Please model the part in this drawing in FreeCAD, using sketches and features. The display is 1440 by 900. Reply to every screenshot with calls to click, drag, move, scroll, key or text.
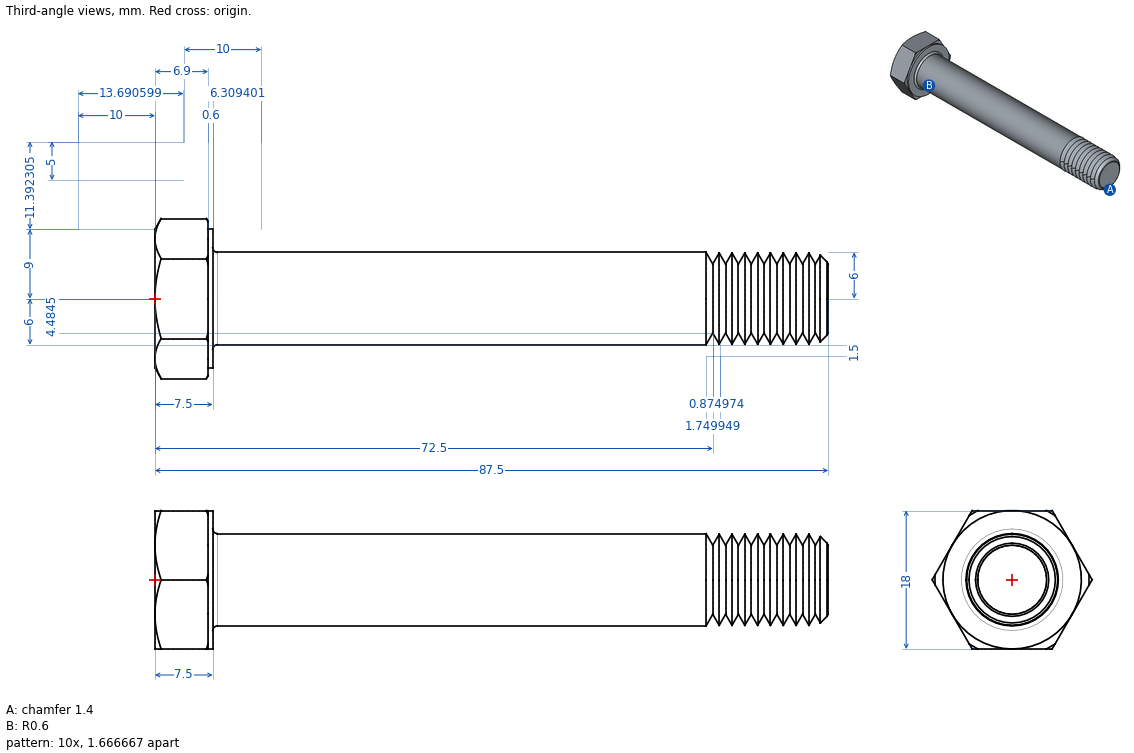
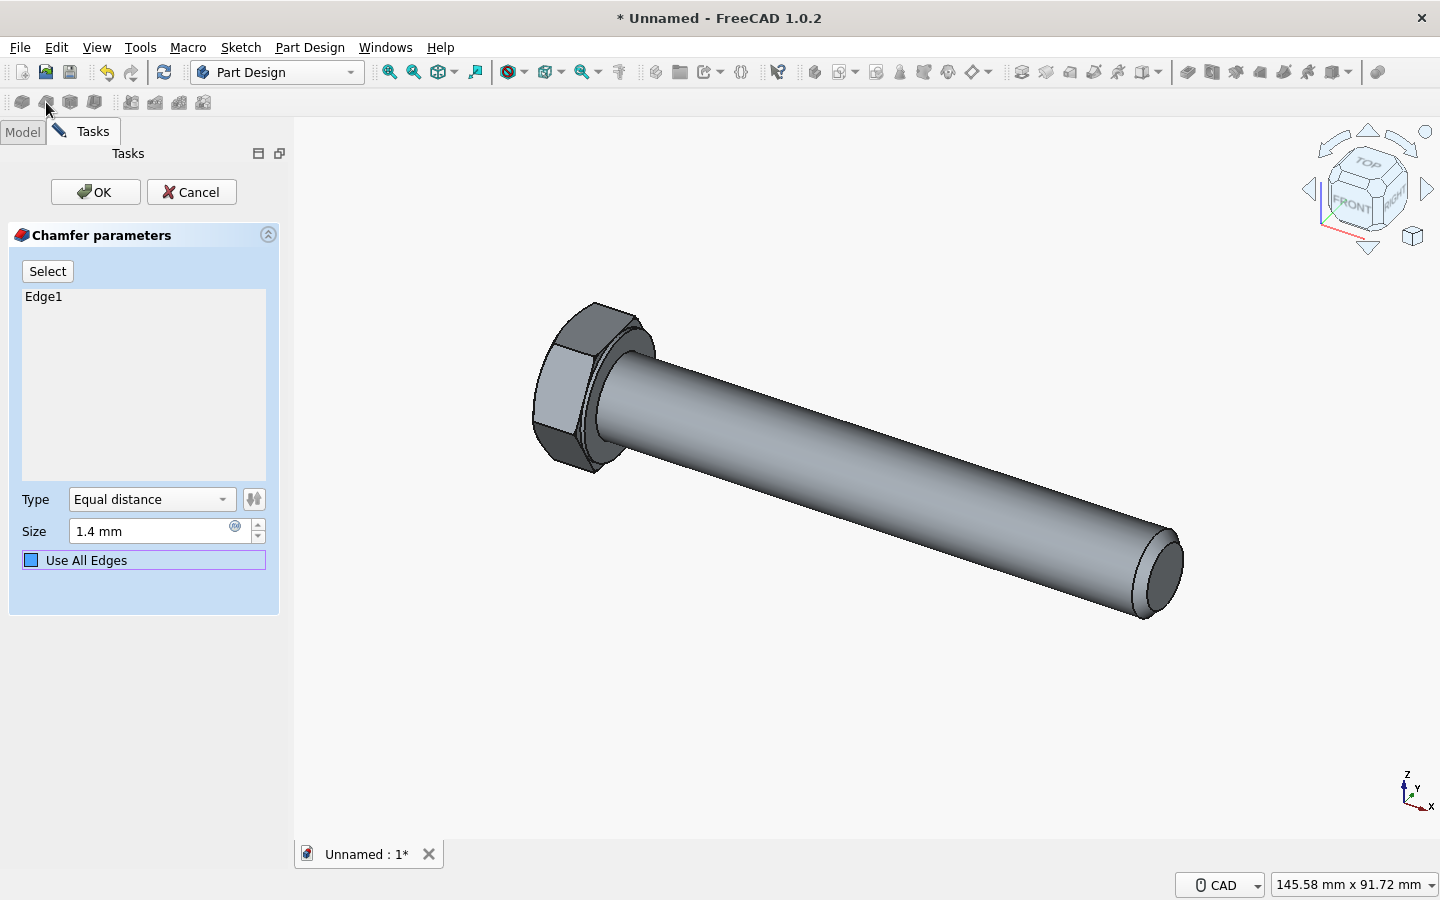
click(96, 192)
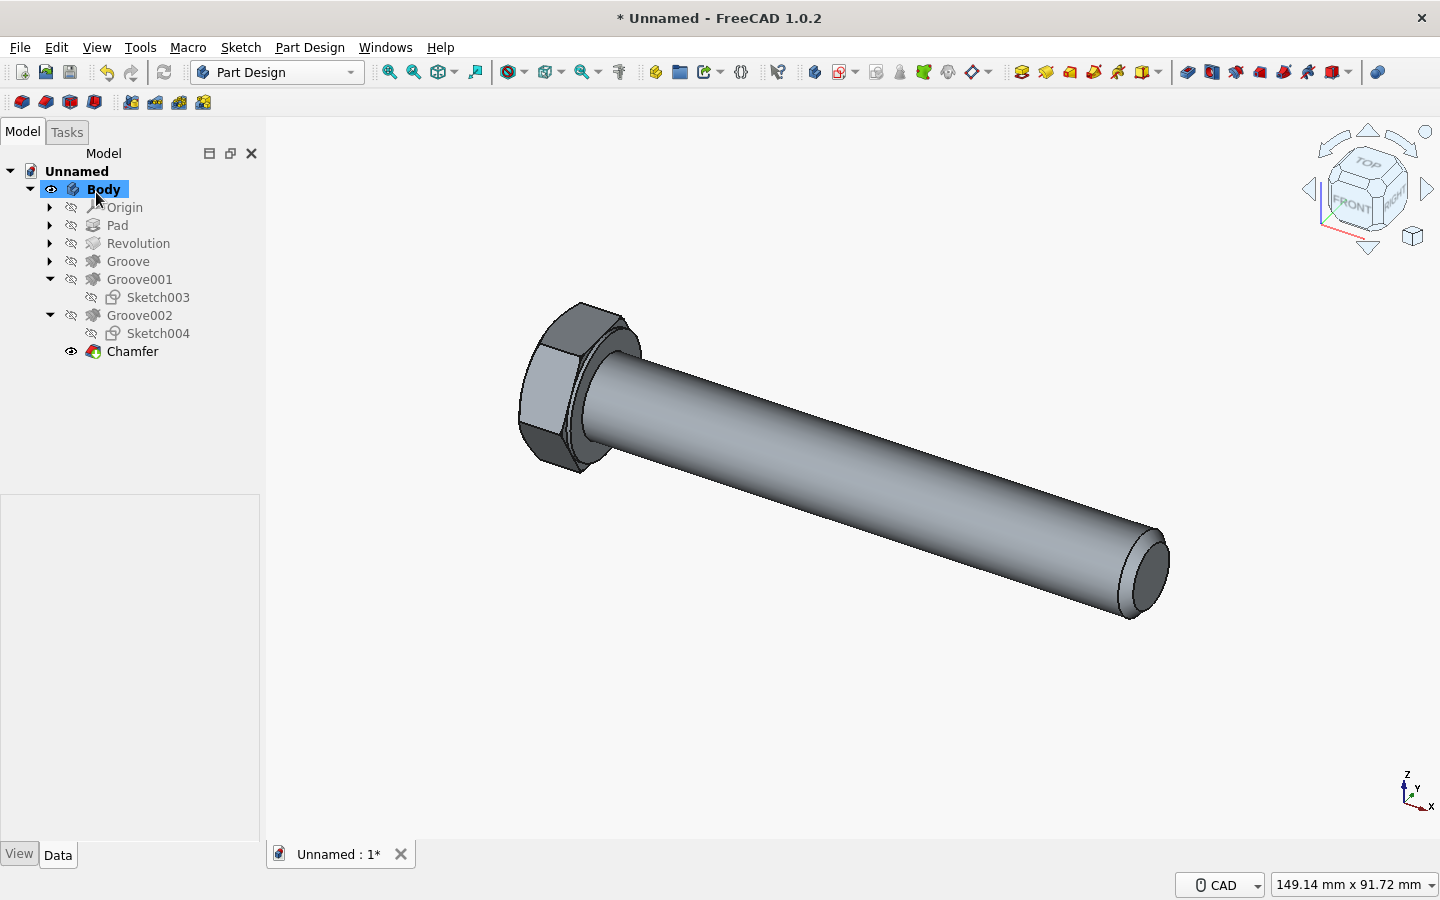
key(0)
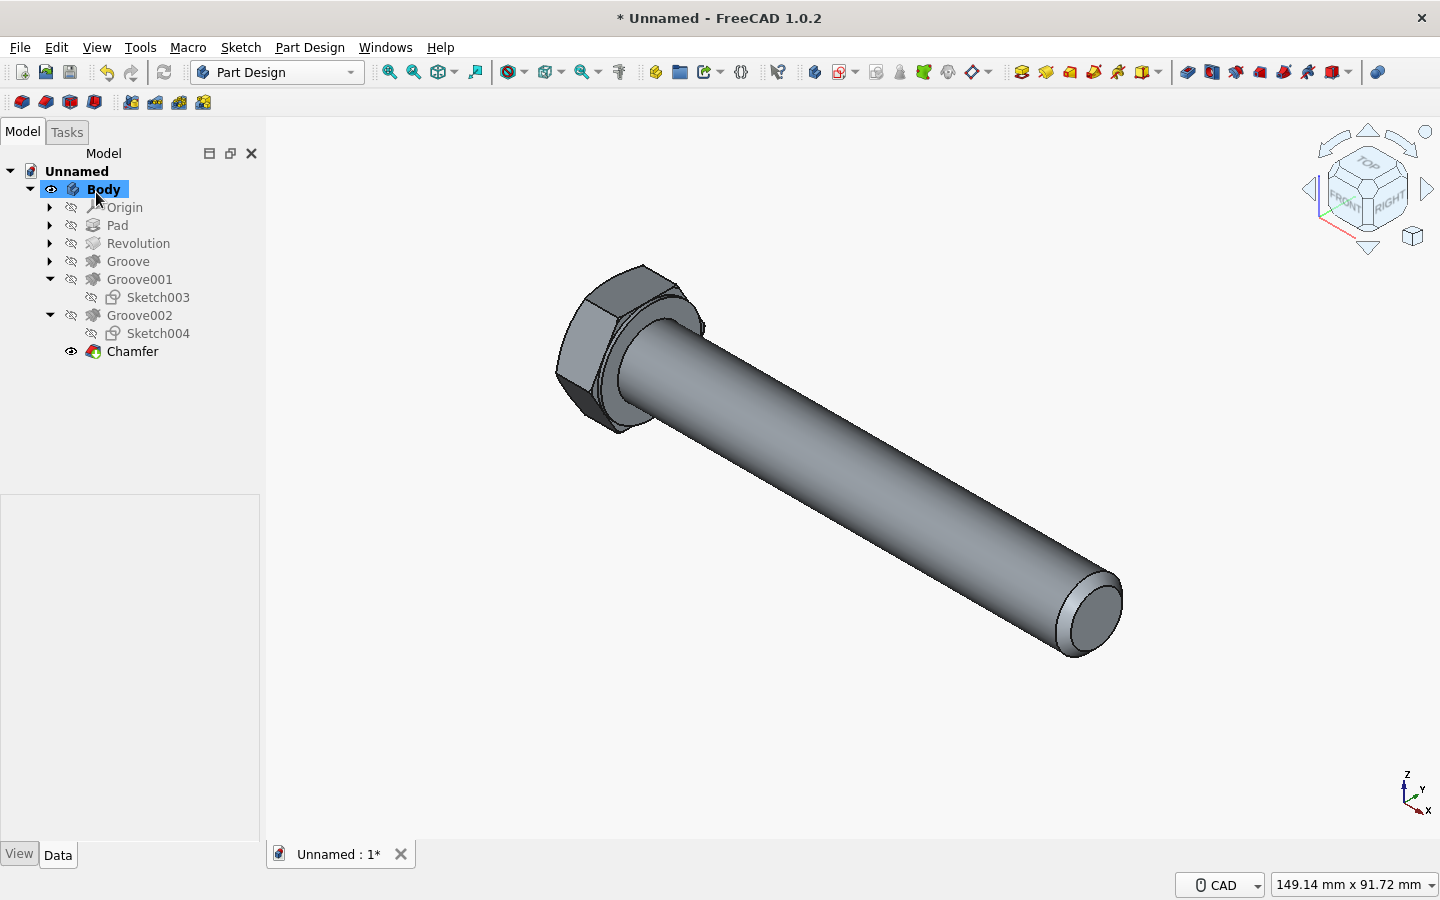
key(2)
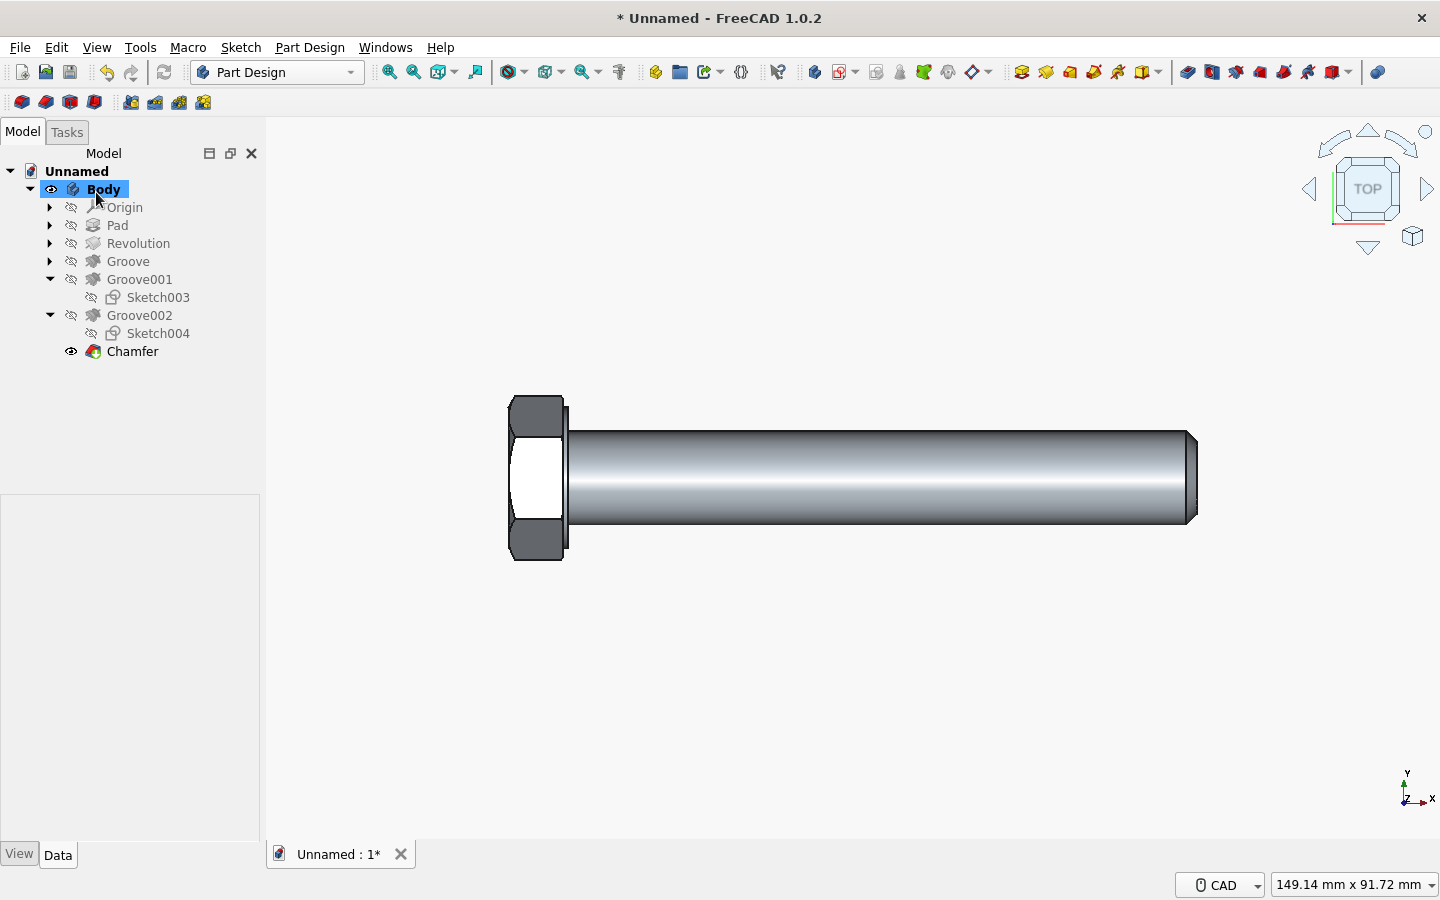
key(1)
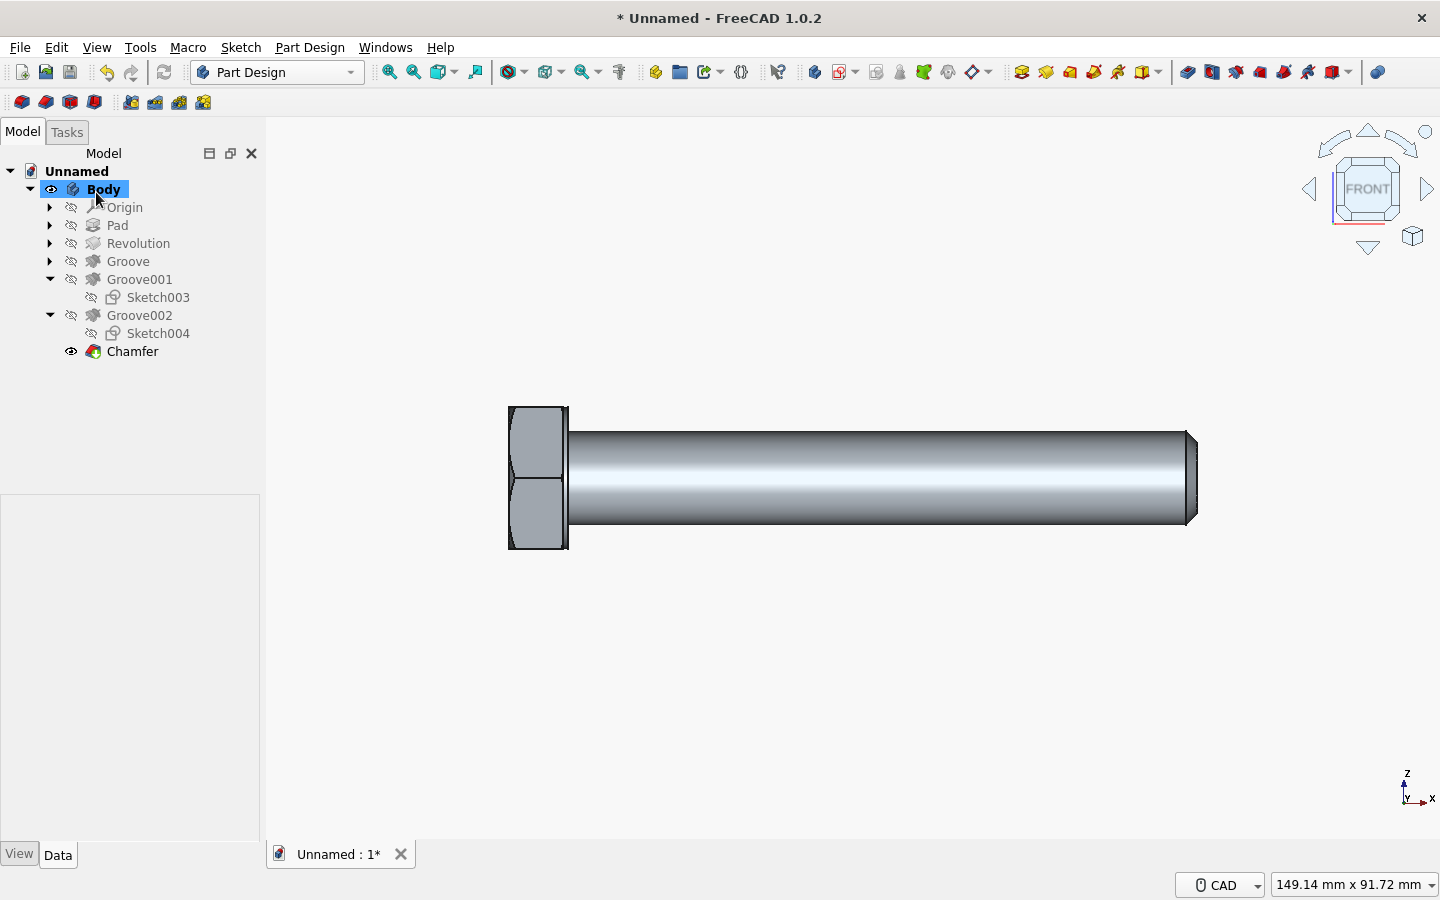
key(3)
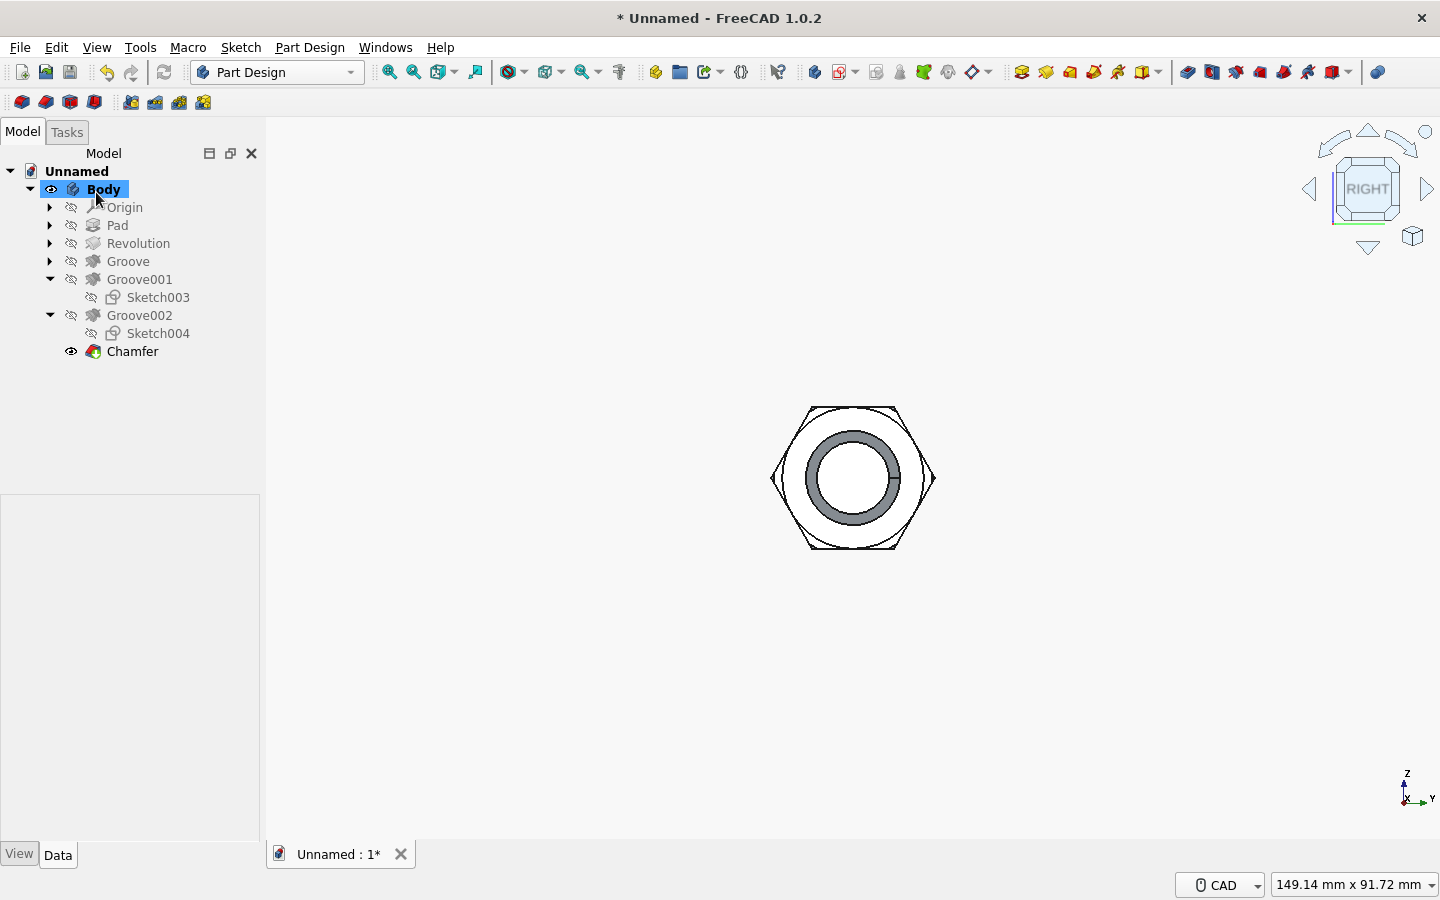
click(390, 72)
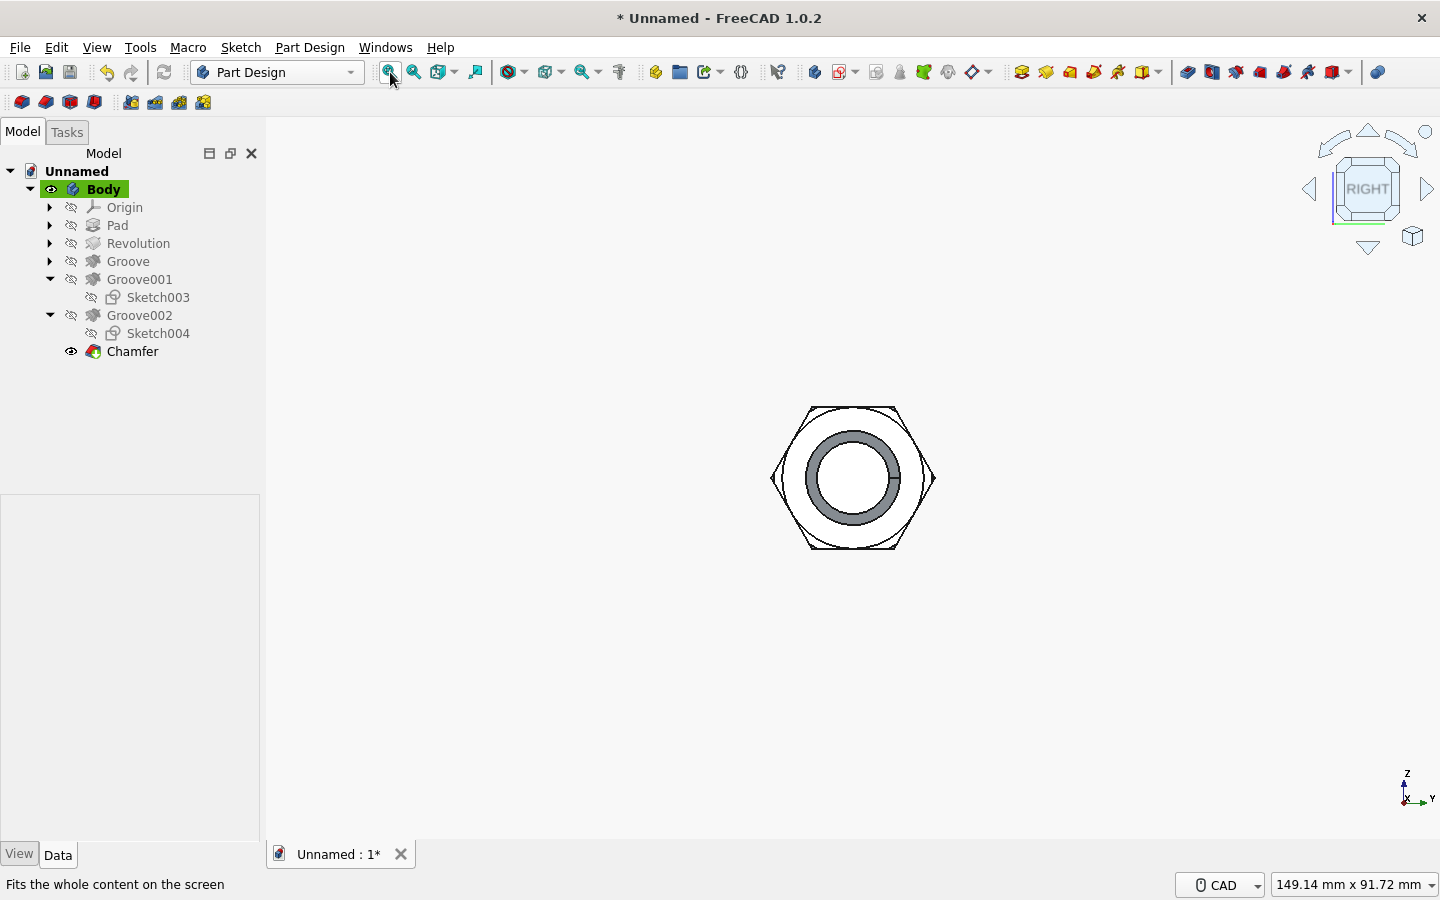
key(5)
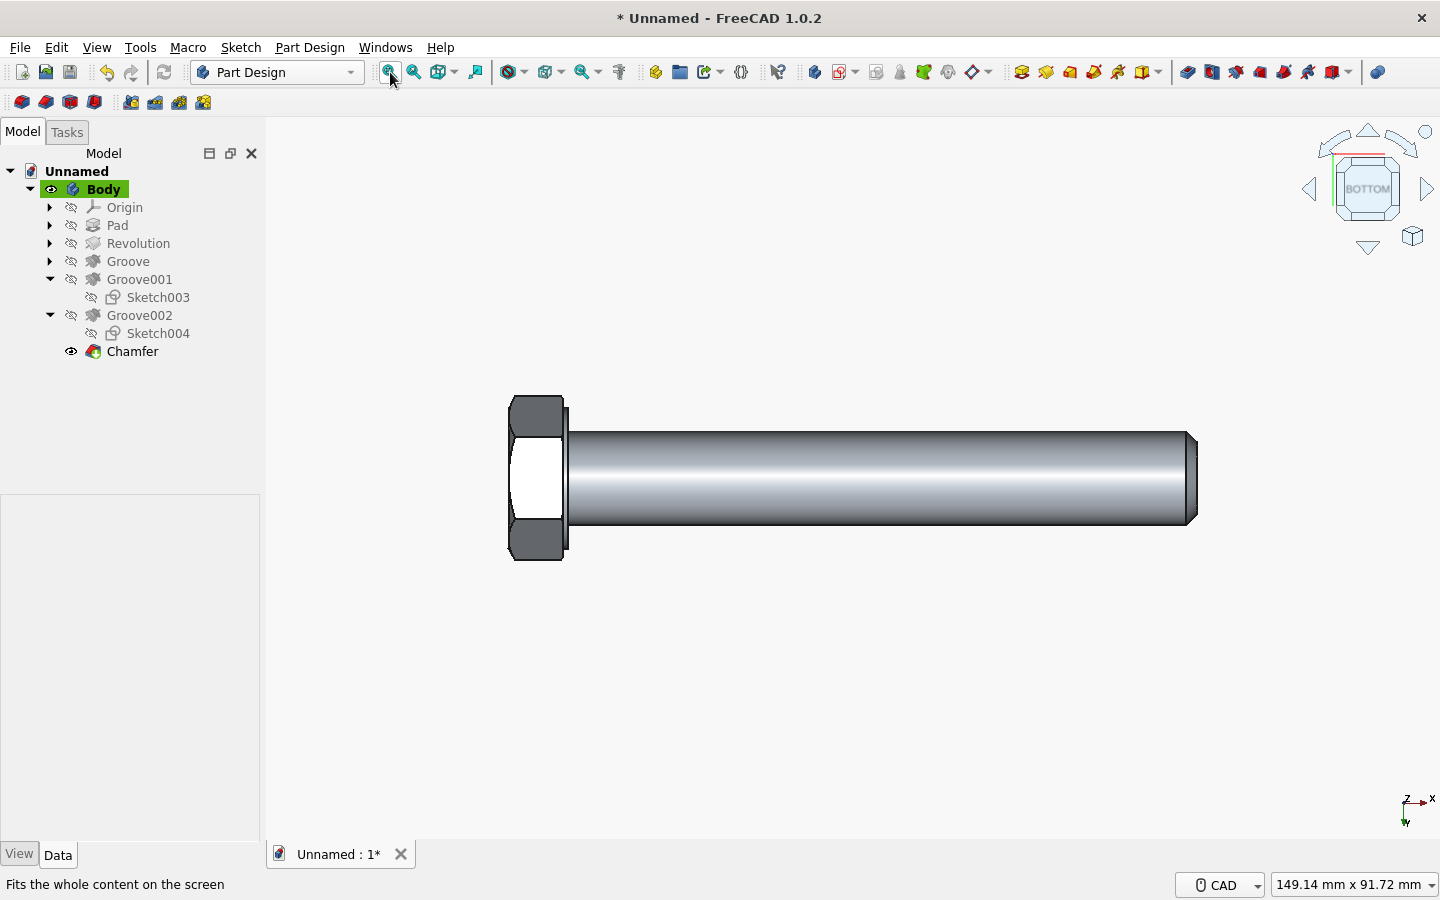
key(4)